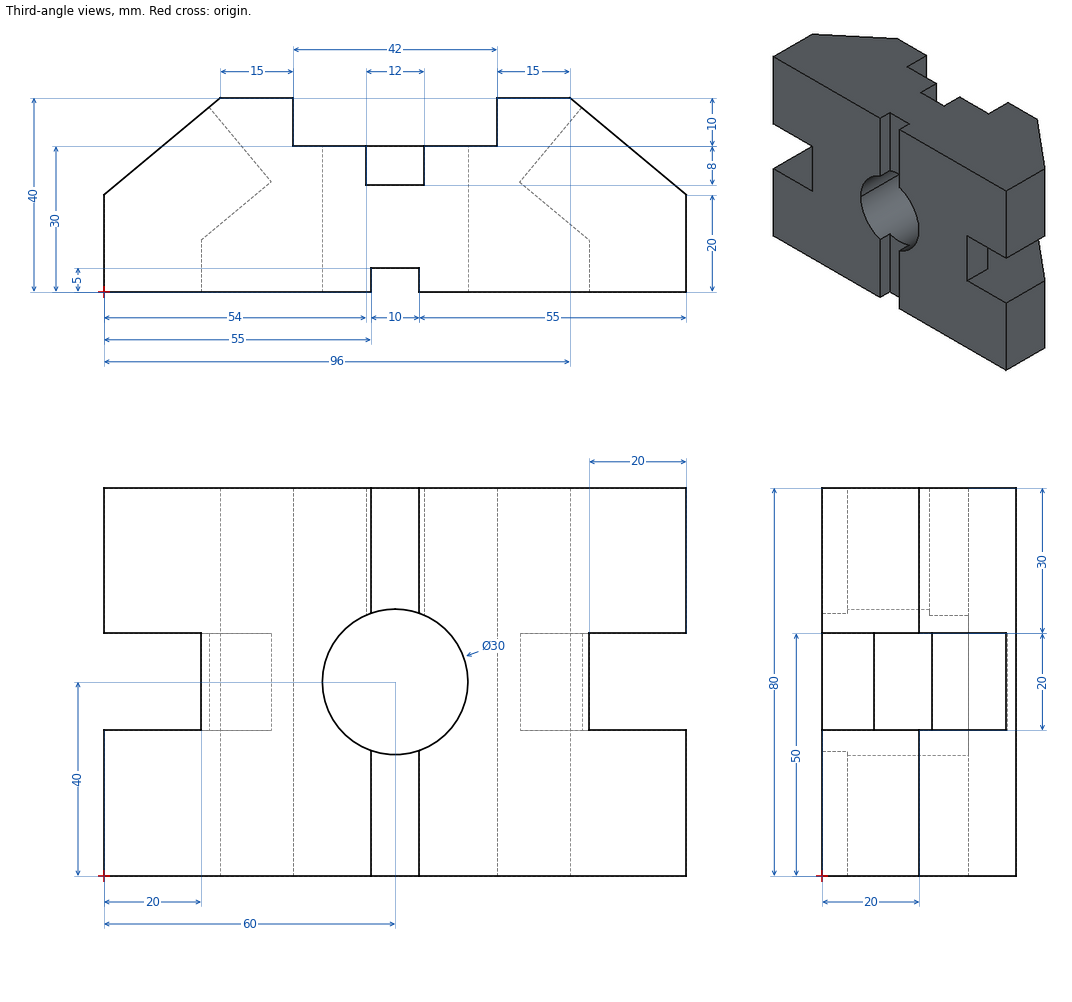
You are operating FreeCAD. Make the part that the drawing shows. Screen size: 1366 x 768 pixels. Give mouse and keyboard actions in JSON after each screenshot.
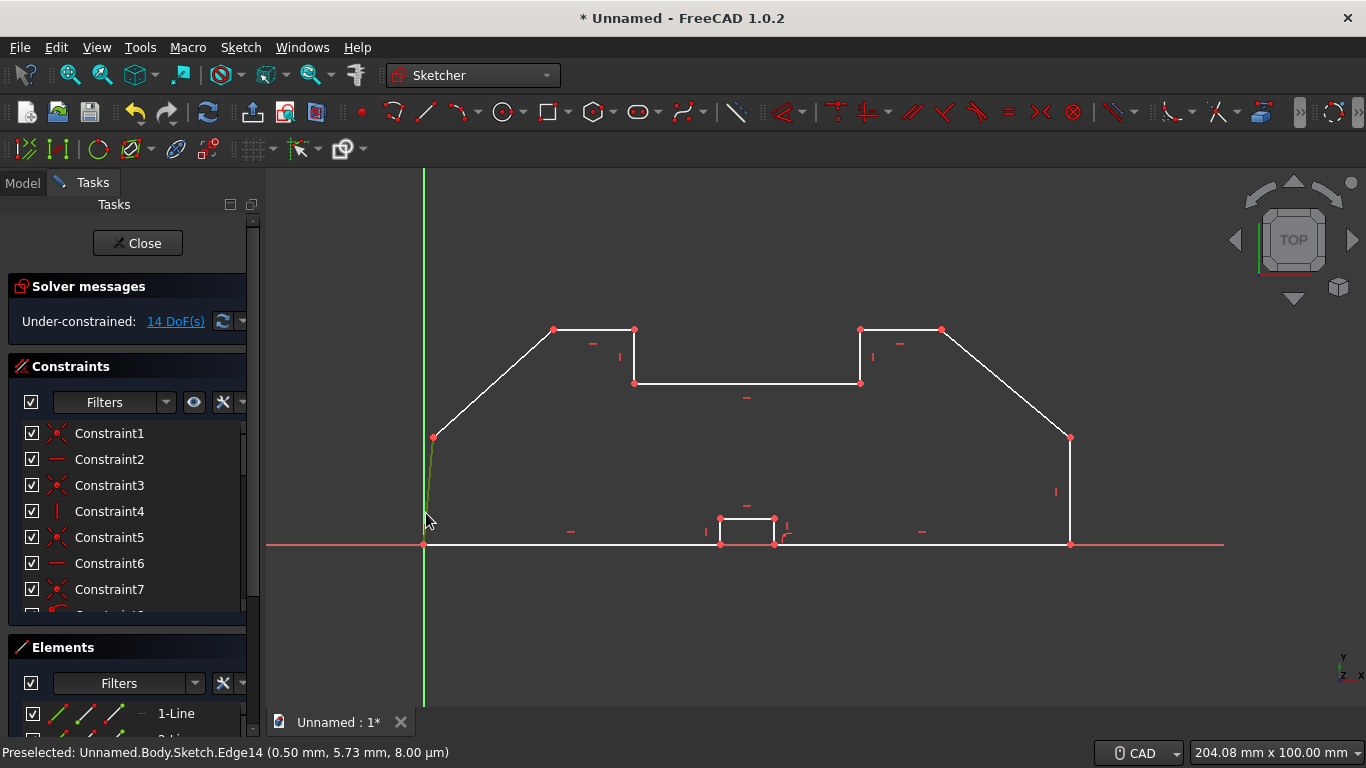
{"action": "key", "text": "v"}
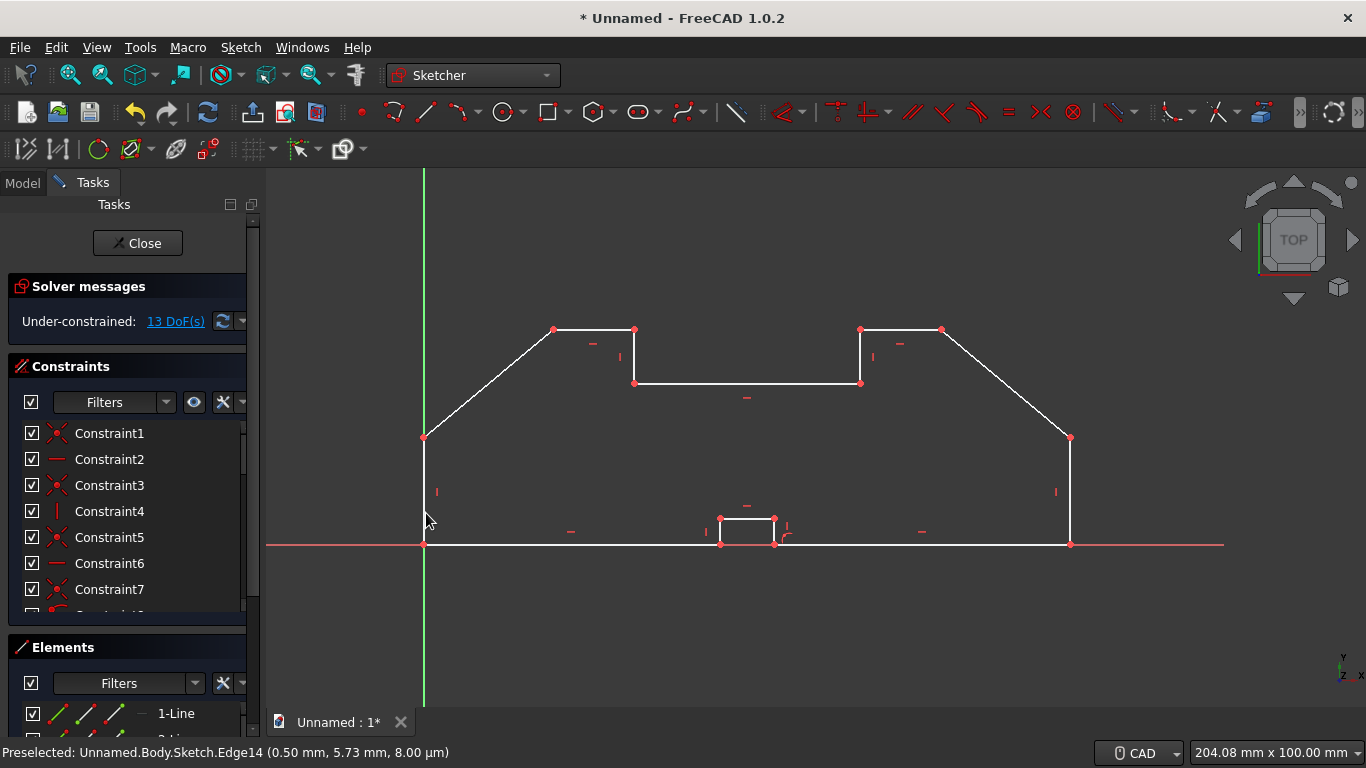
{"action": "left_click", "coordinate": [782, 112]}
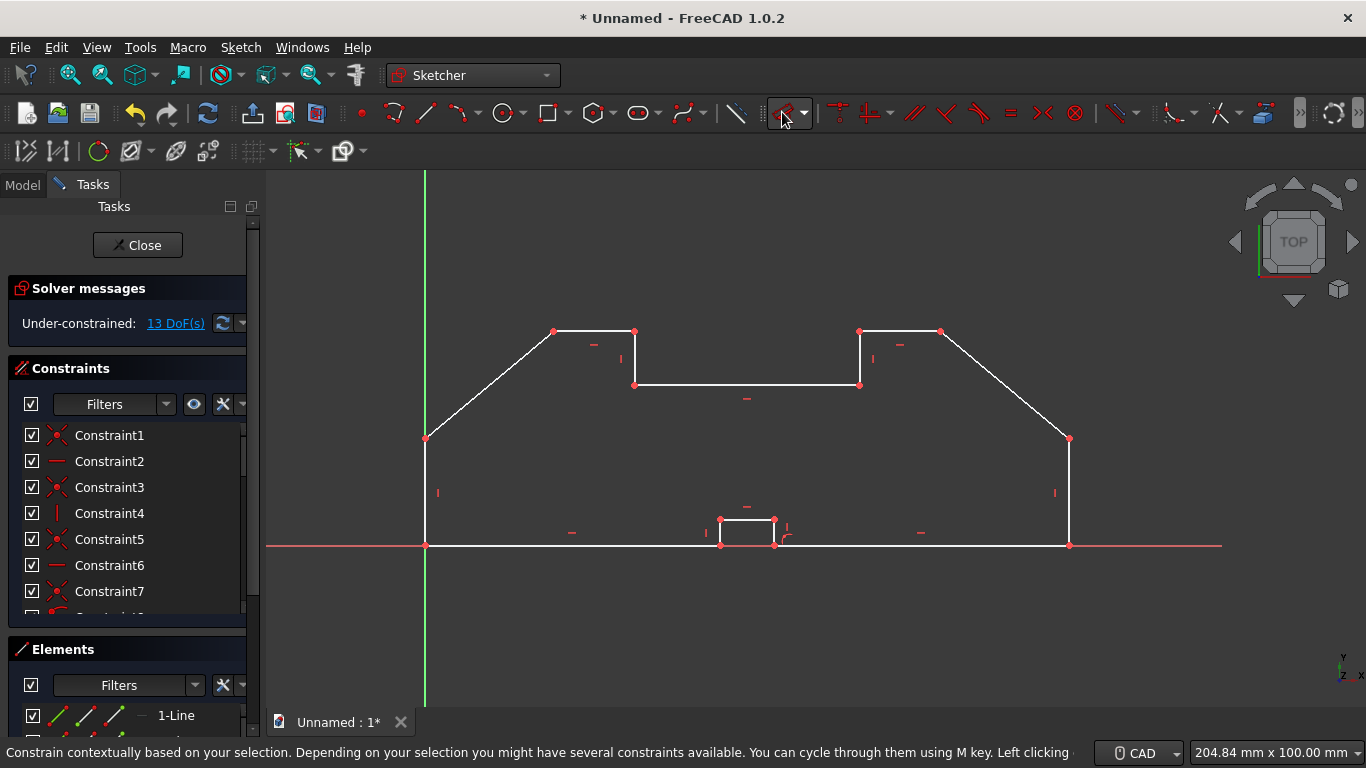
{"action": "scroll", "coordinate": [720, 535], "scroll_direction": "up", "scroll_amount": 2}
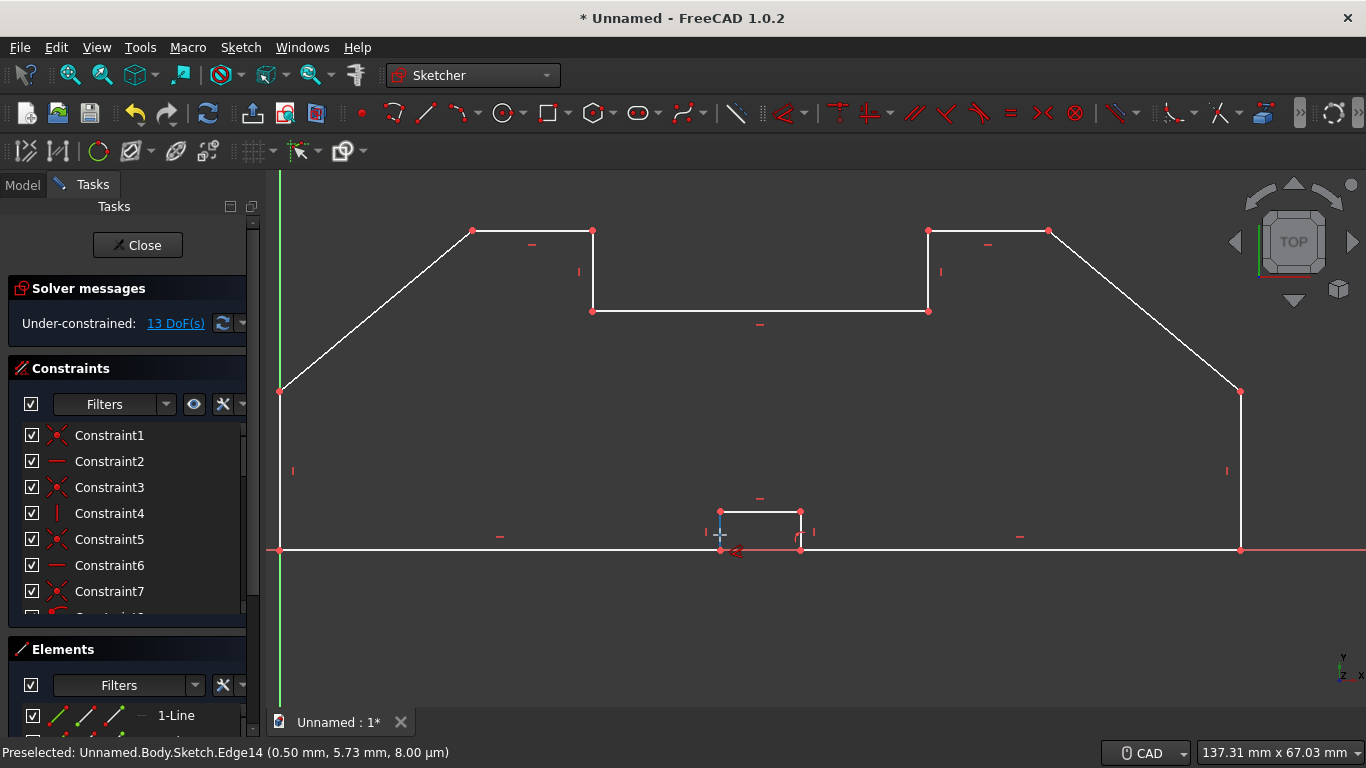
{"action": "left_click", "coordinate": [720, 535]}
{"action": "left_click", "coordinate": [686, 531]}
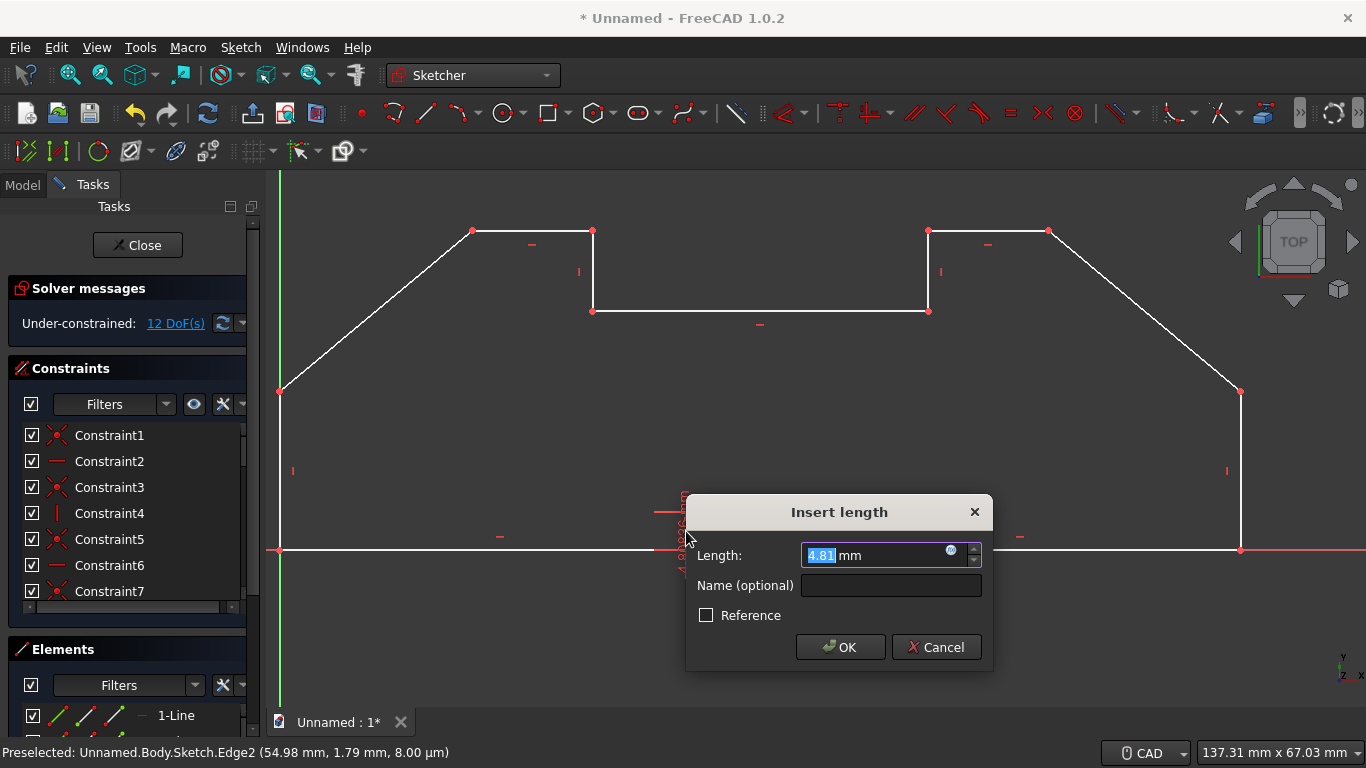
{"action": "type", "text": "5"}
{"action": "key", "text": "Return"}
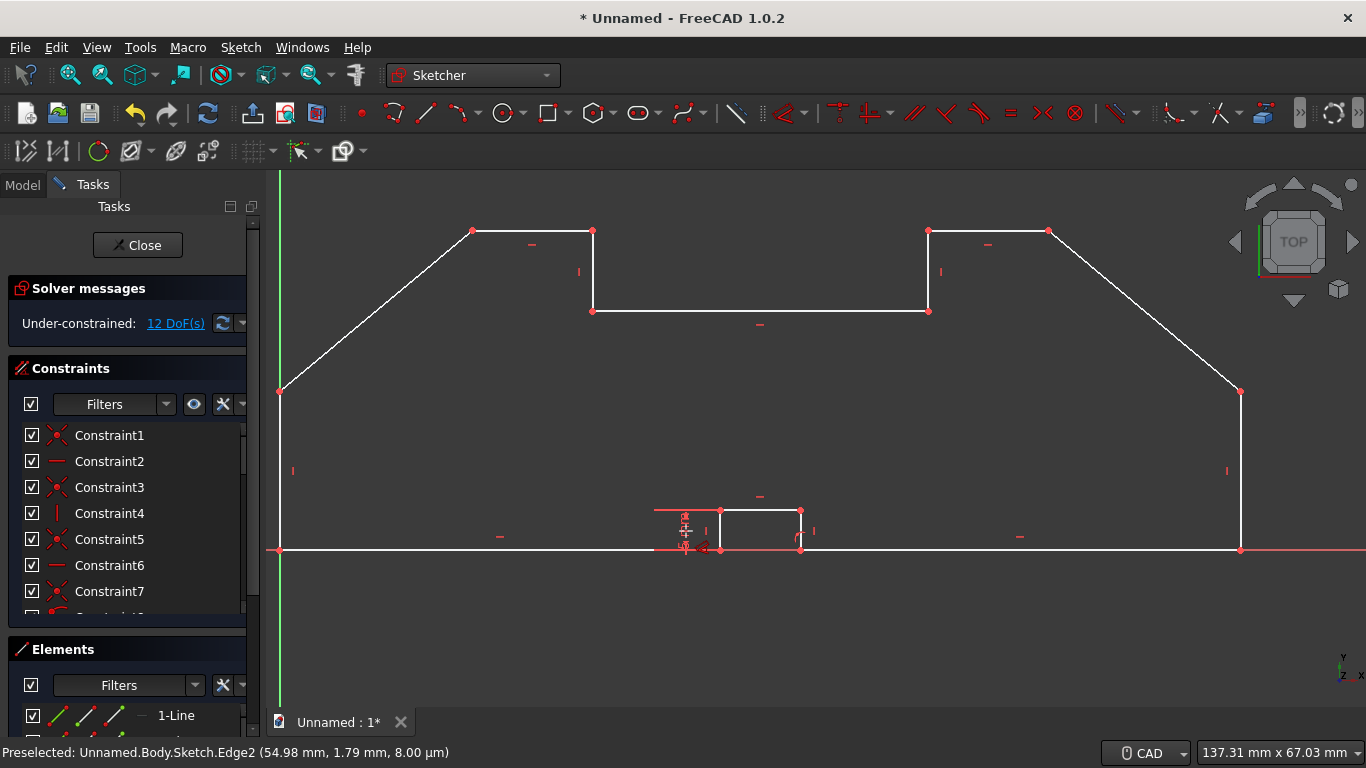
{"action": "left_click", "coordinate": [412, 550]}
{"action": "left_click", "coordinate": [507, 584]}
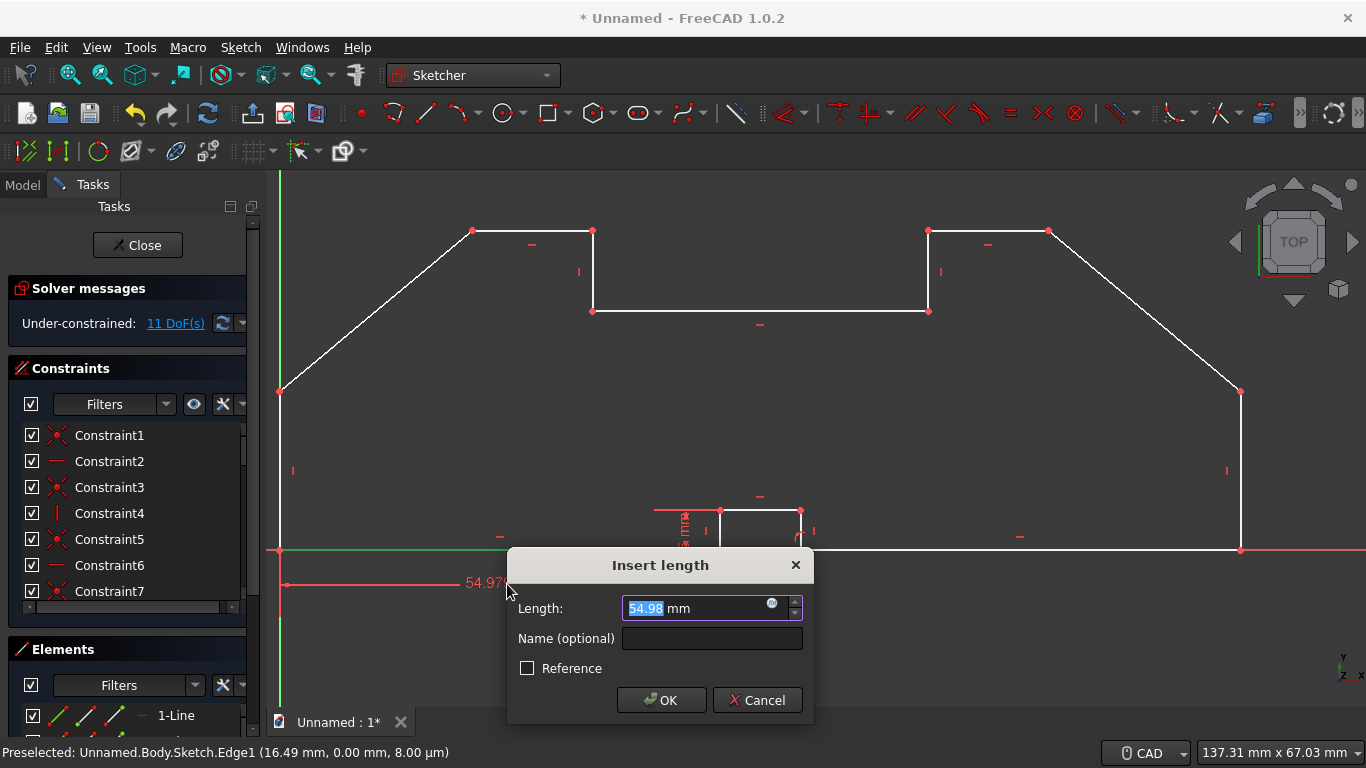
{"action": "type", "text": "55"}
{"action": "key", "text": "Return"}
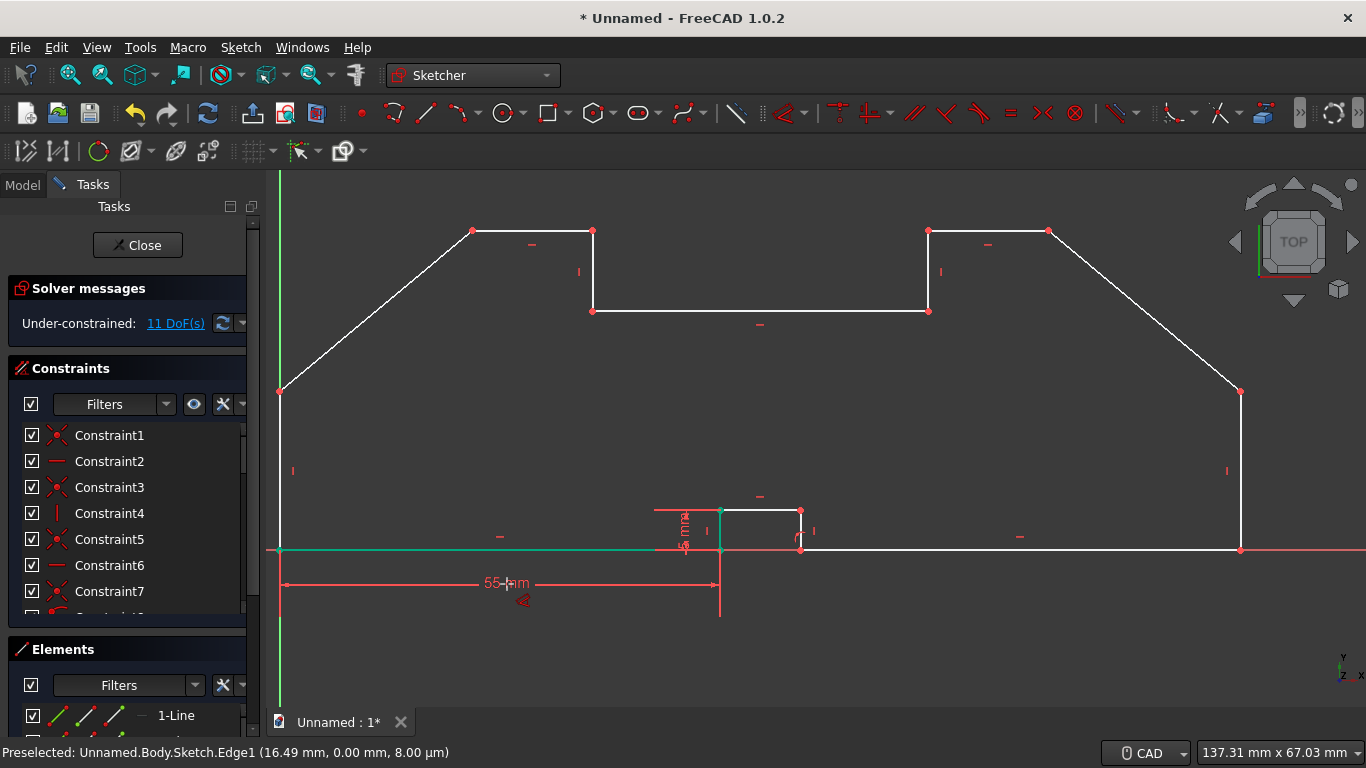
{"action": "left_click", "coordinate": [745, 510]}
{"action": "left_click", "coordinate": [761, 476]}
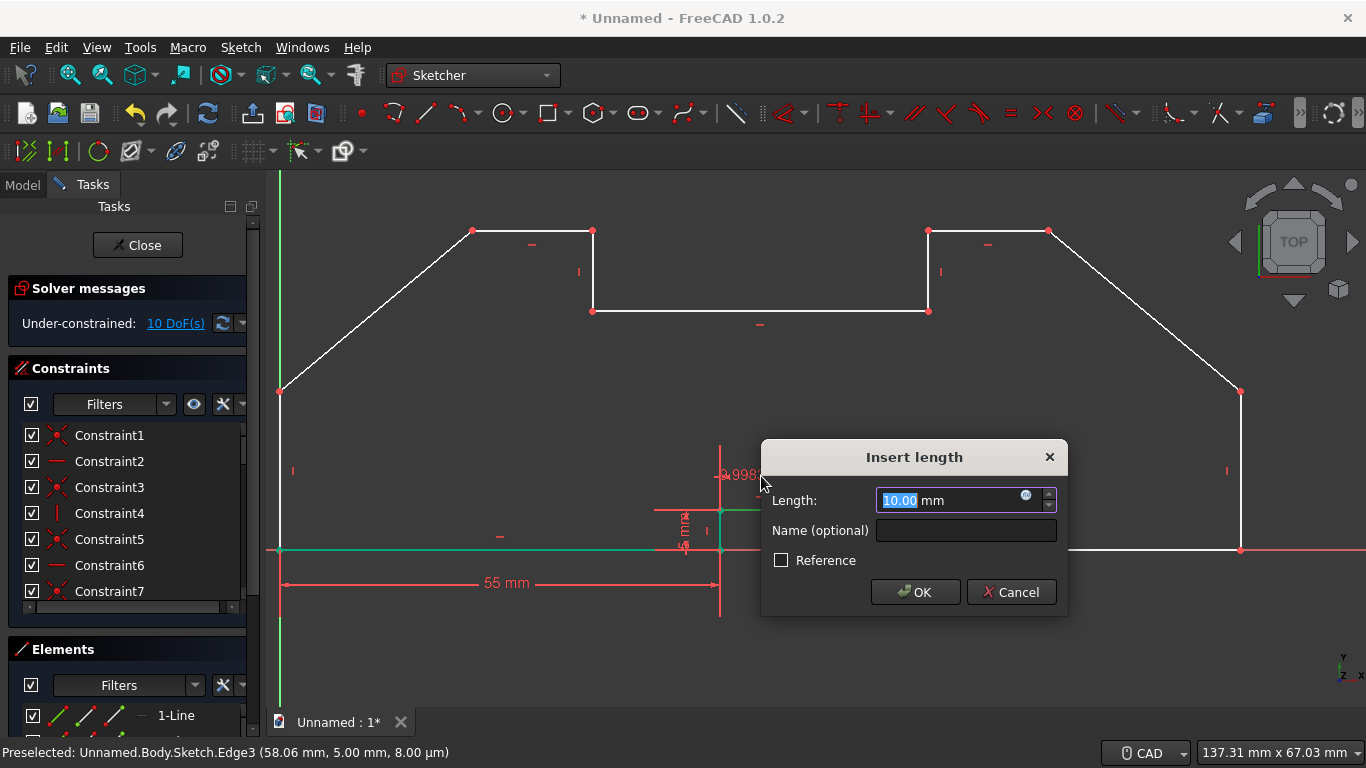
{"action": "type", "text": "10"}
{"action": "key", "text": "Return"}